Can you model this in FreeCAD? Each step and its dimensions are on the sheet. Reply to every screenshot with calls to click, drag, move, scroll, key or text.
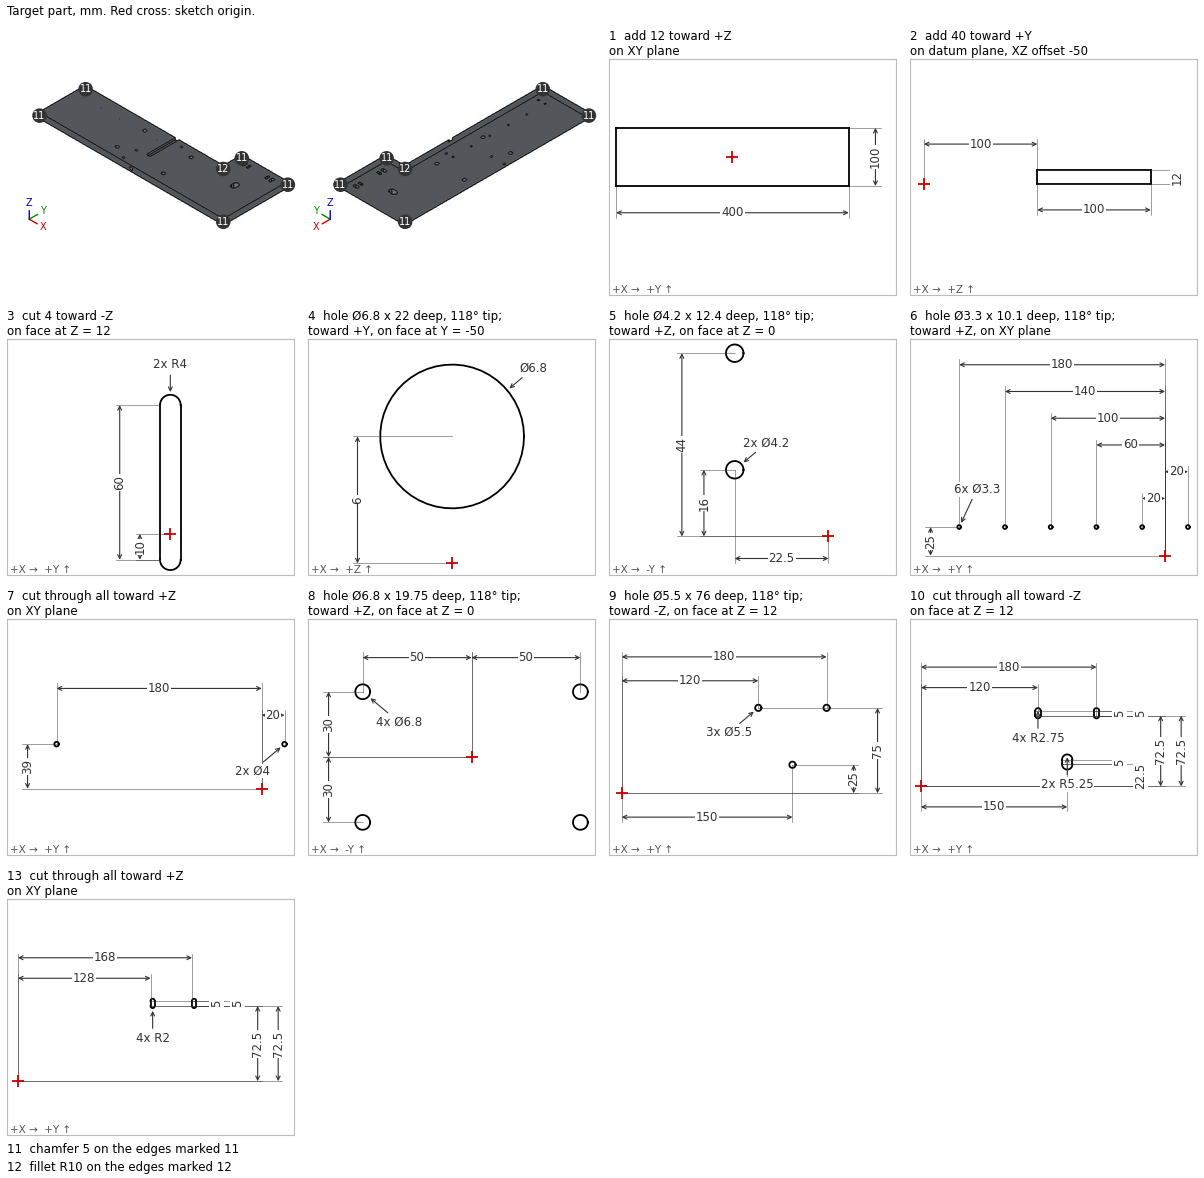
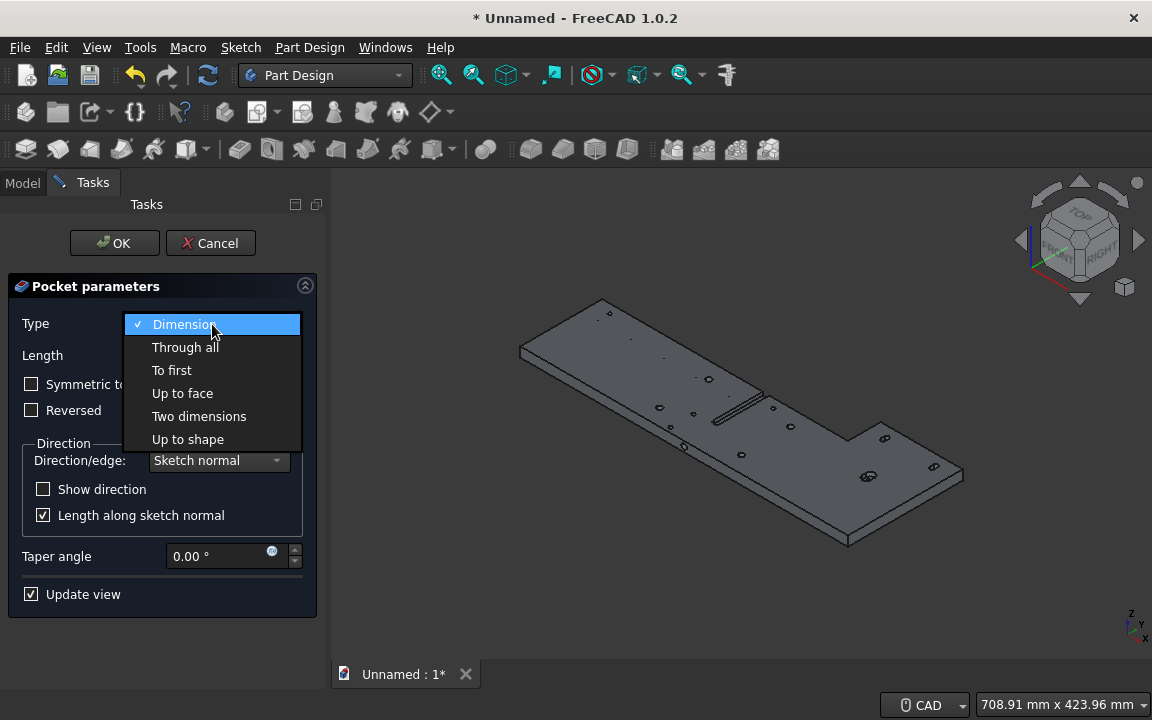
click(212, 348)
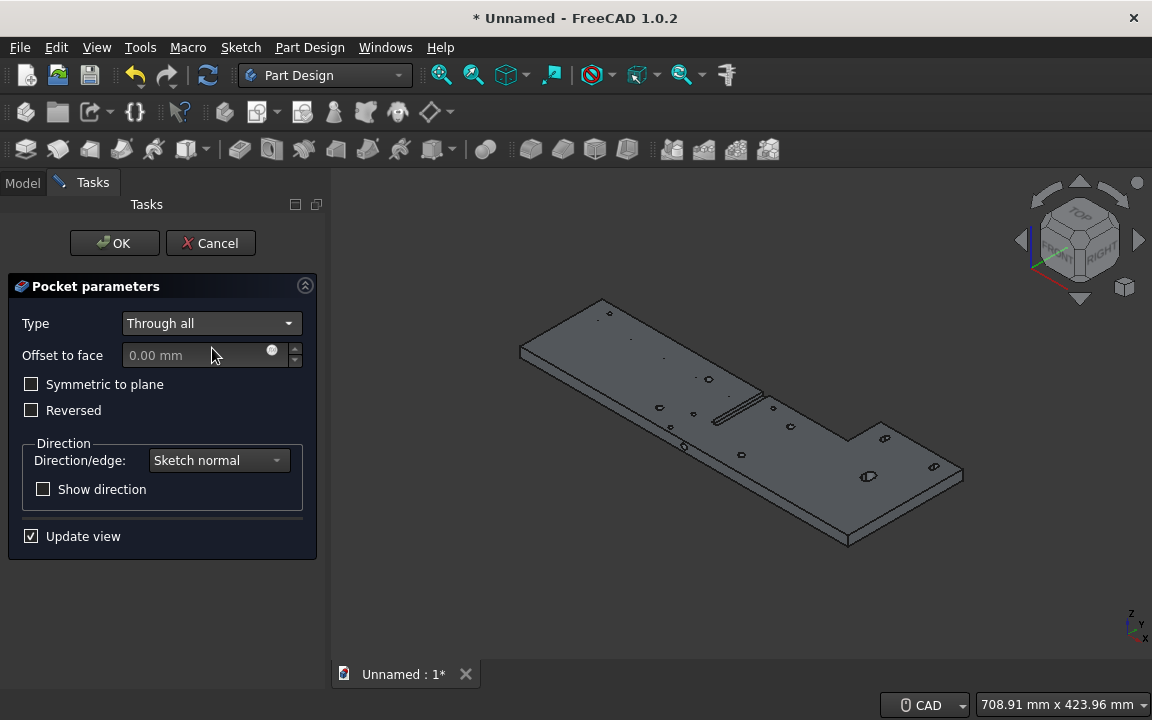
click(115, 243)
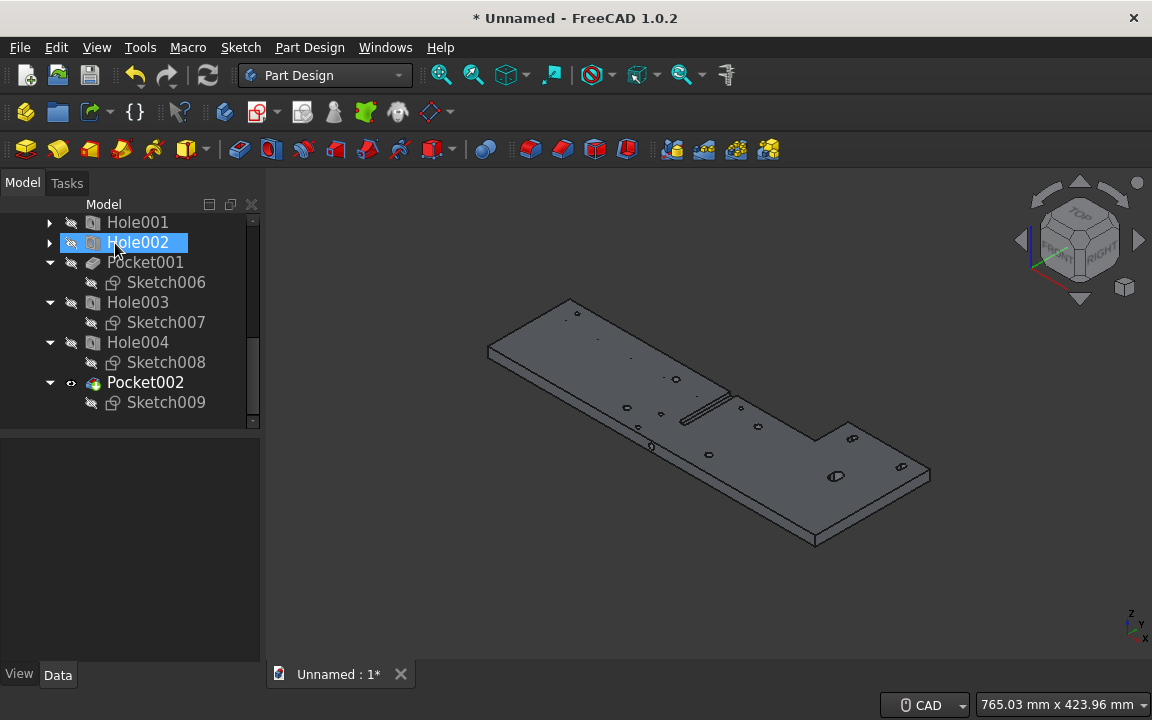
click(815, 541)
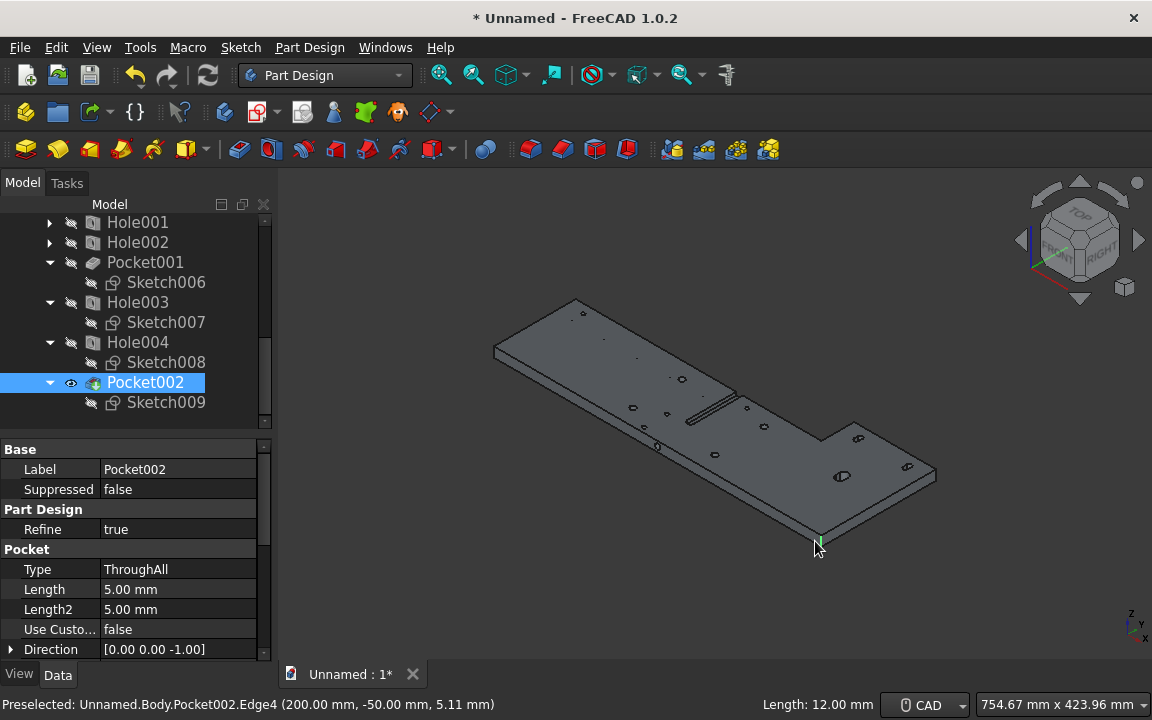
scroll(854, 427, up, 6)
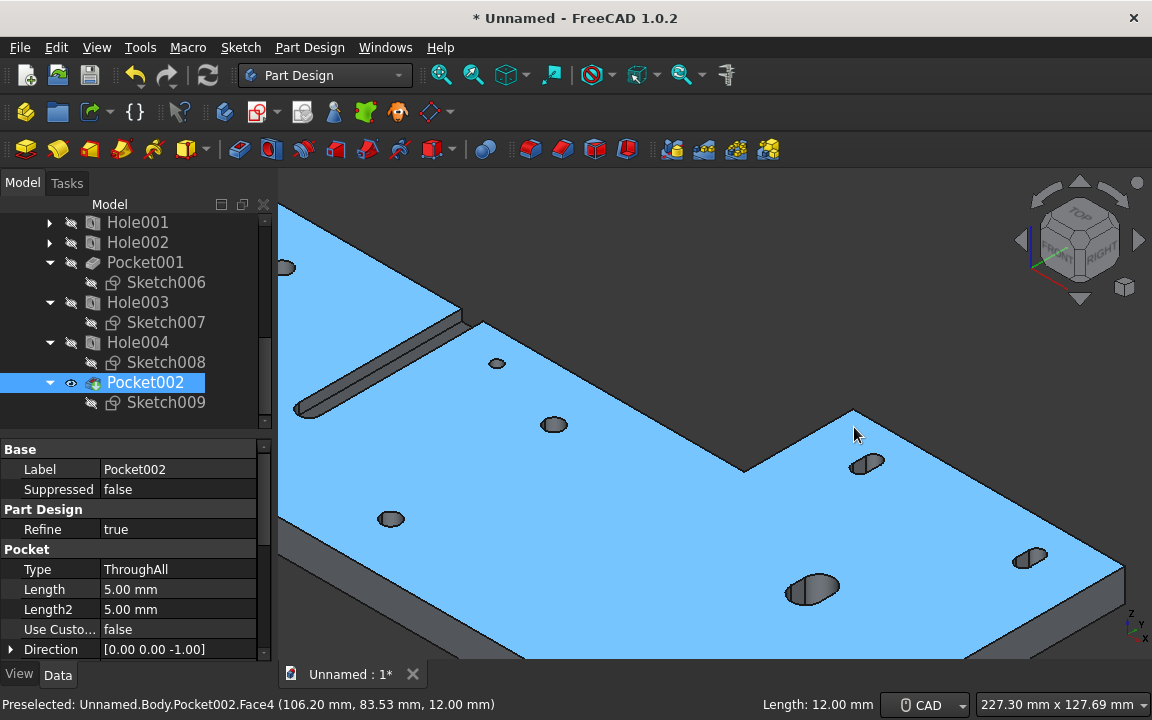
click(442, 76)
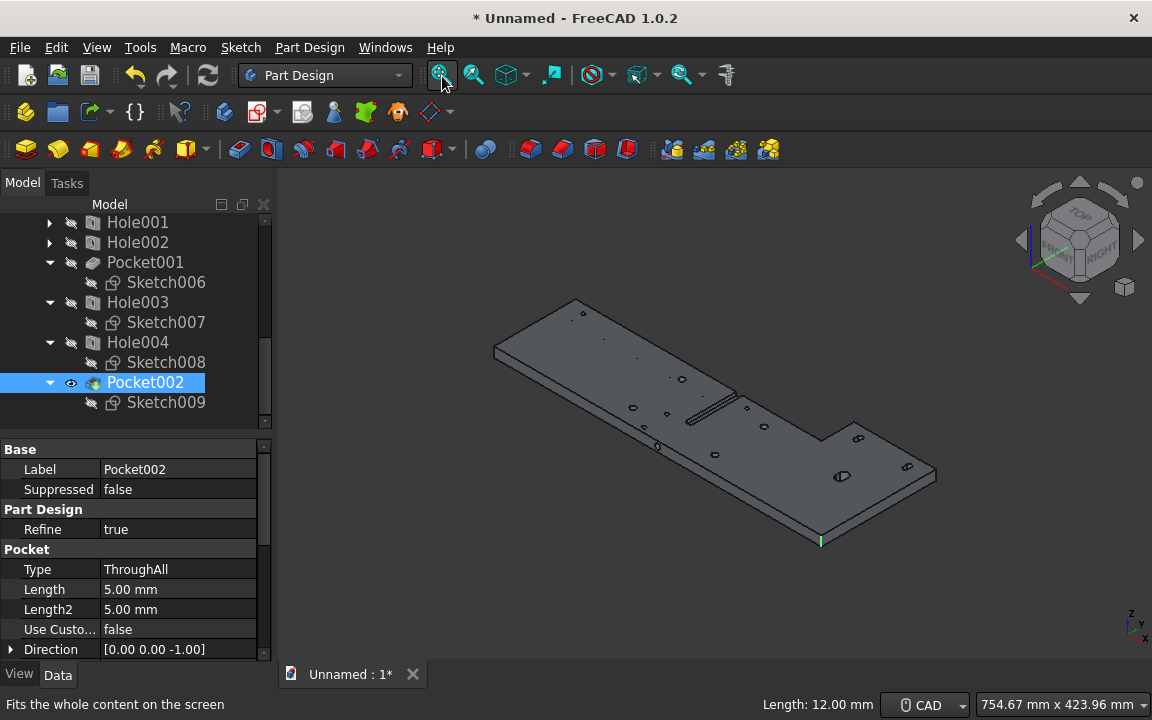
key(2)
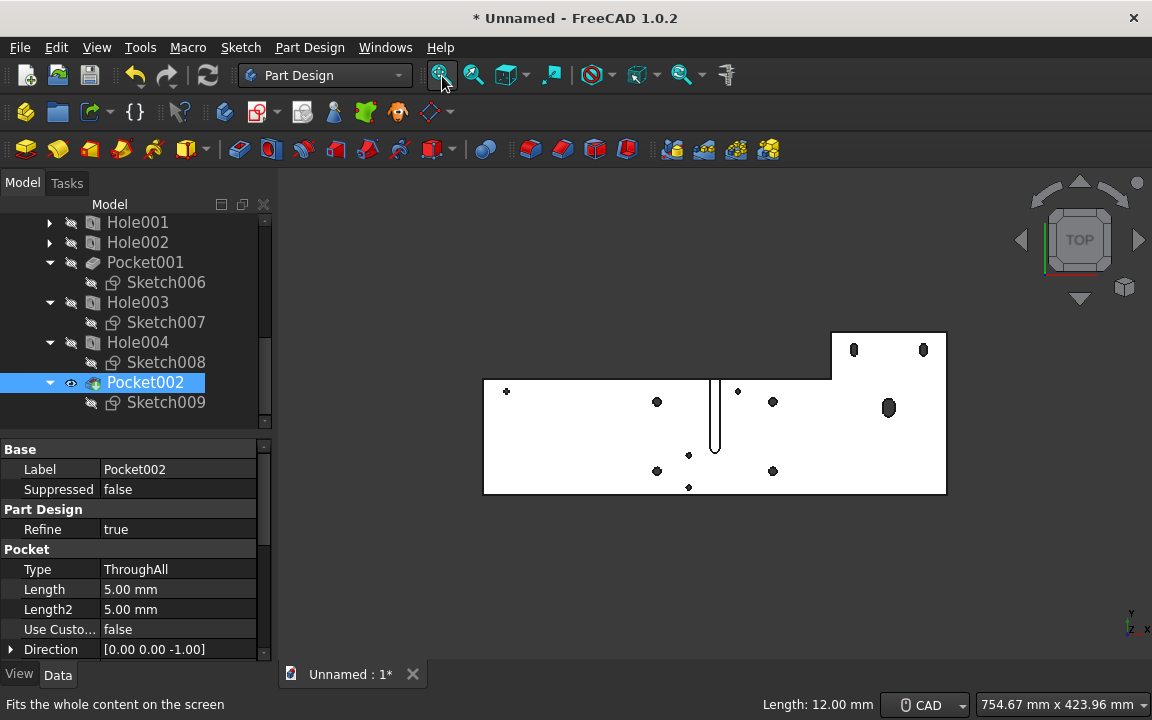
scroll(831, 331, up, 6)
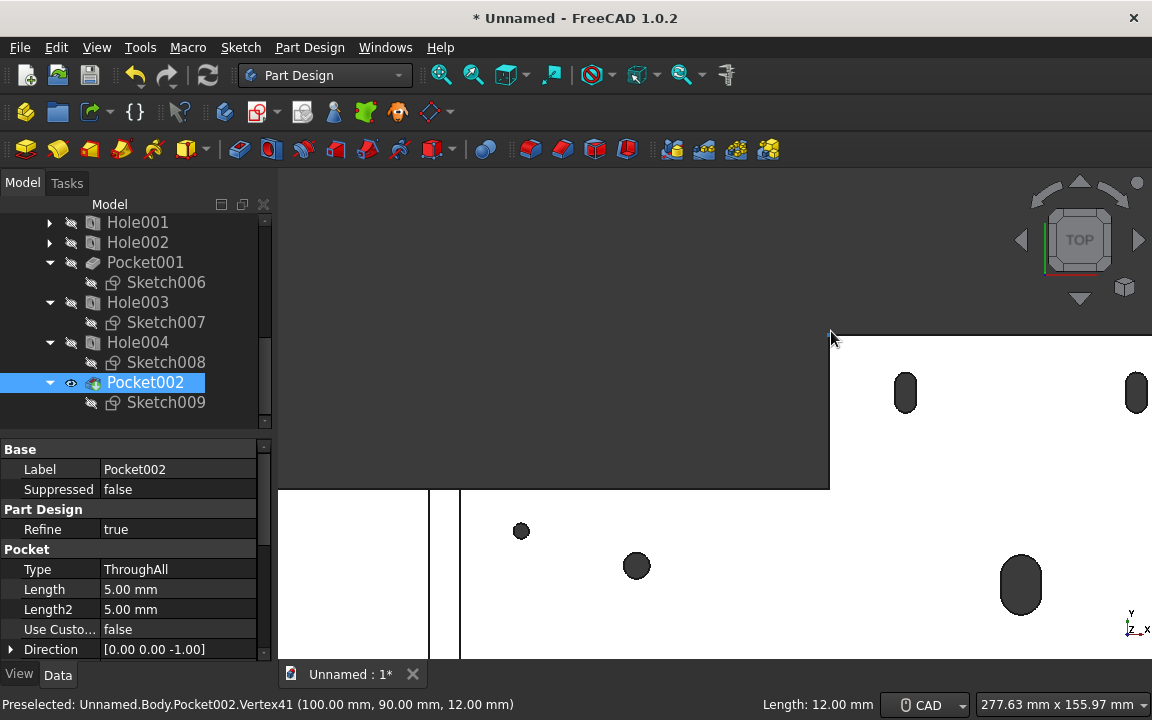
click(442, 76)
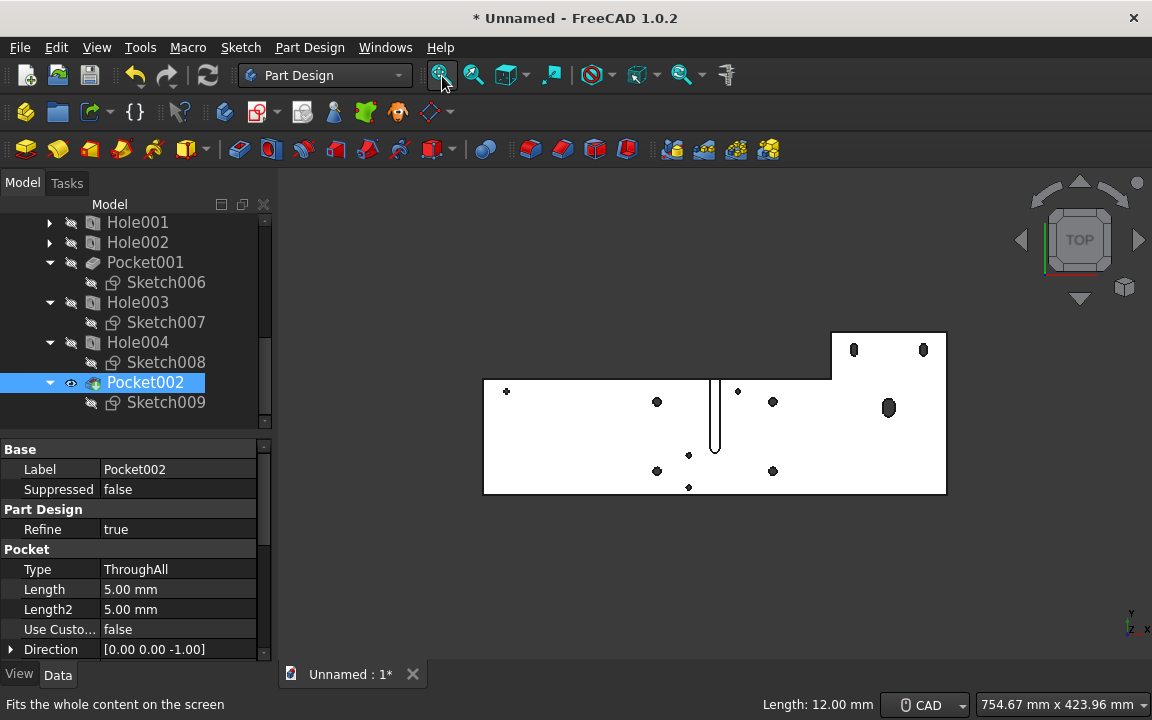
key(0)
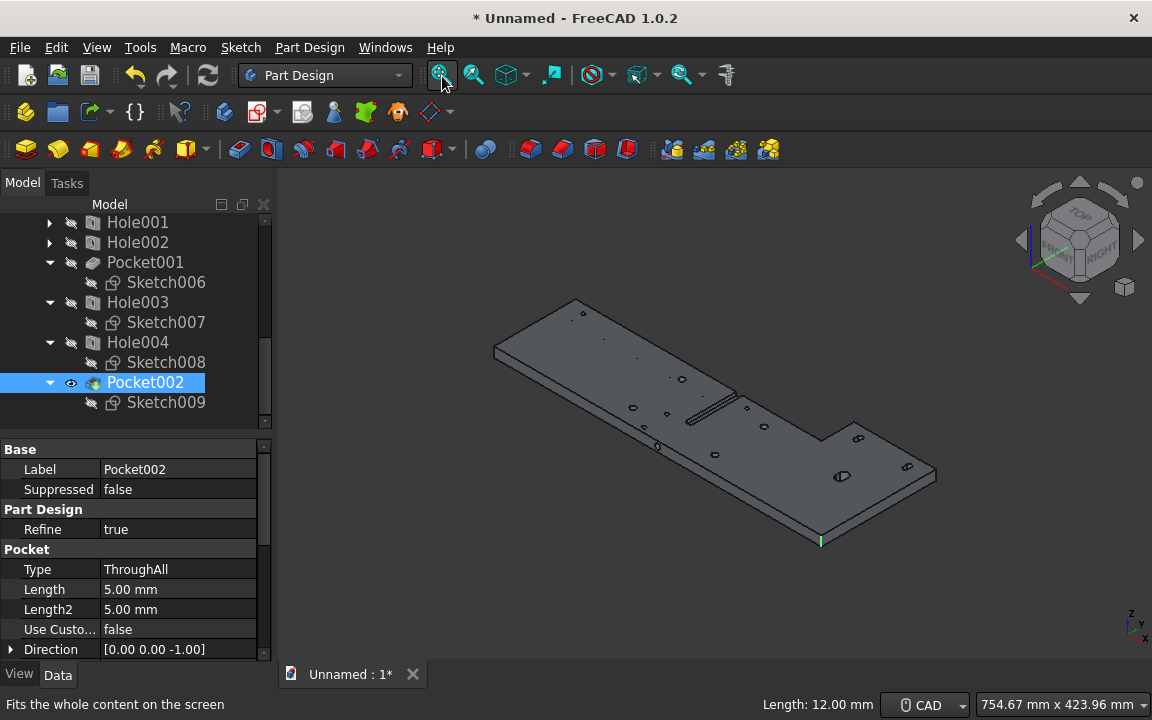
scroll(854, 427, up, 6)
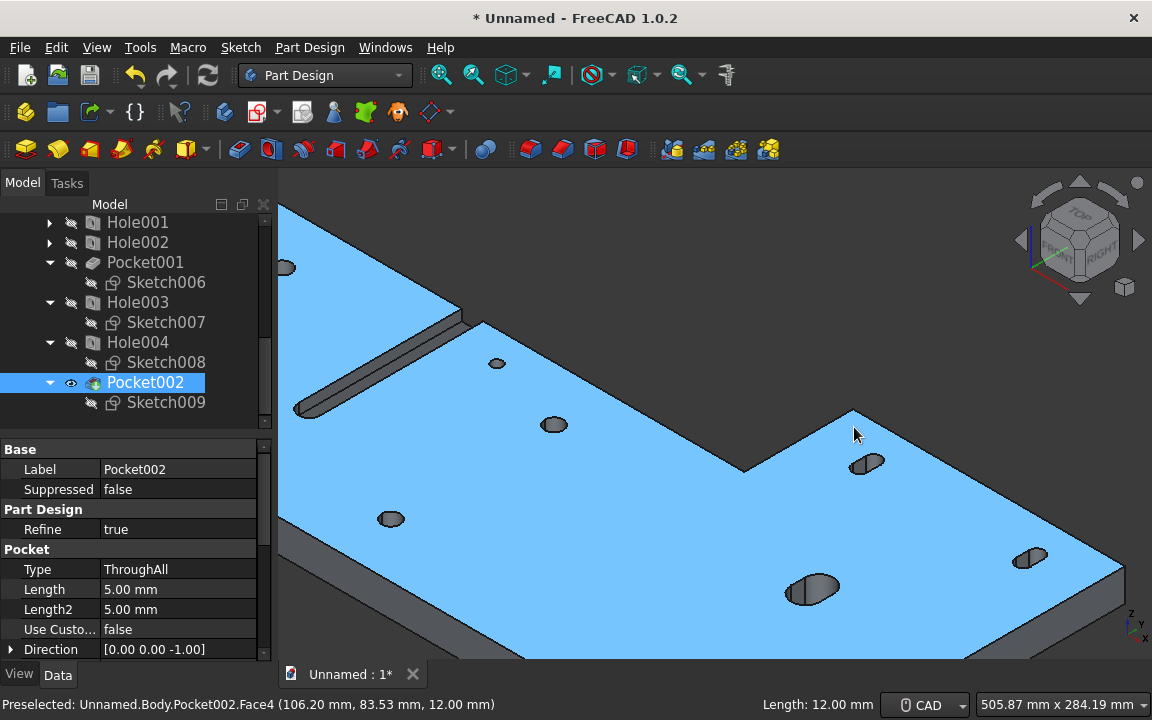
click(442, 76)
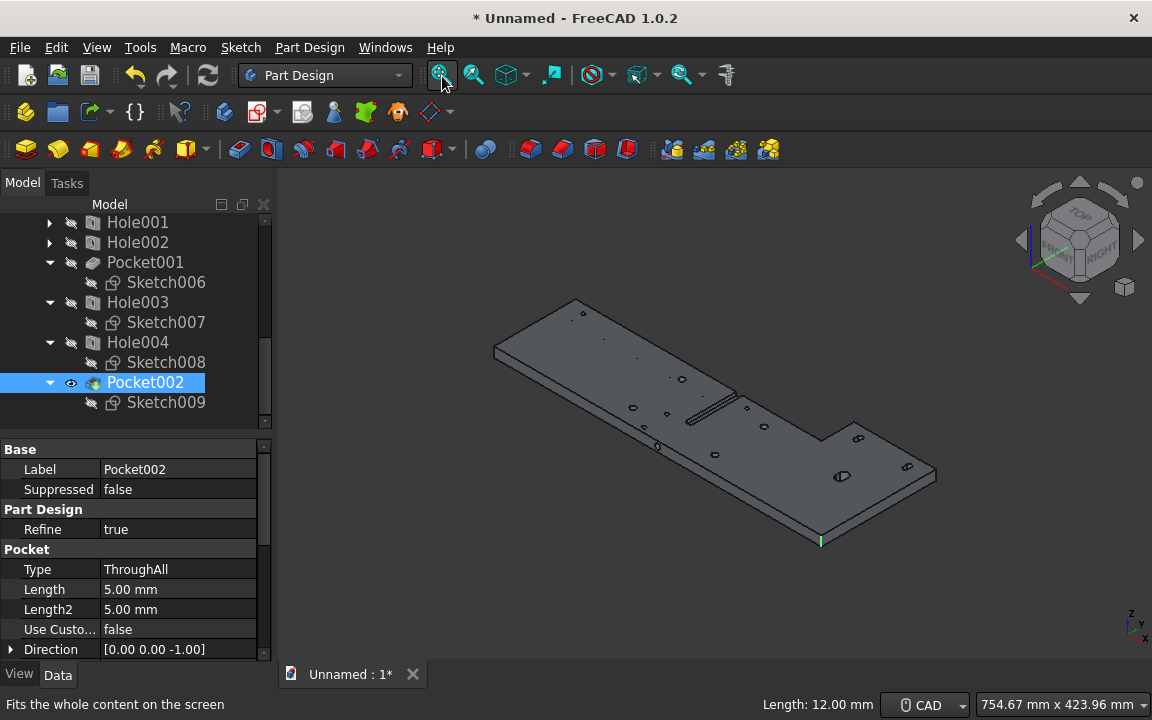
key(1)